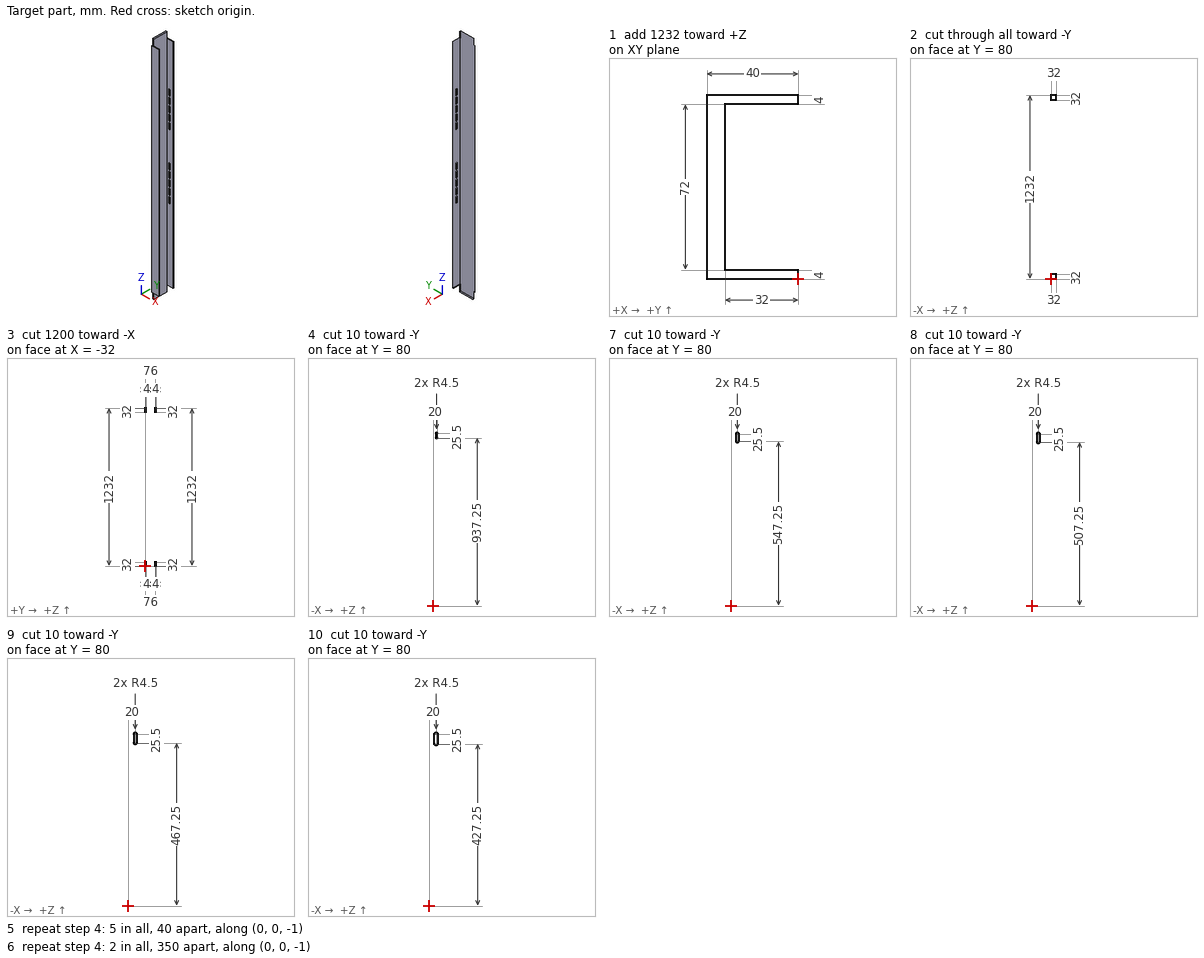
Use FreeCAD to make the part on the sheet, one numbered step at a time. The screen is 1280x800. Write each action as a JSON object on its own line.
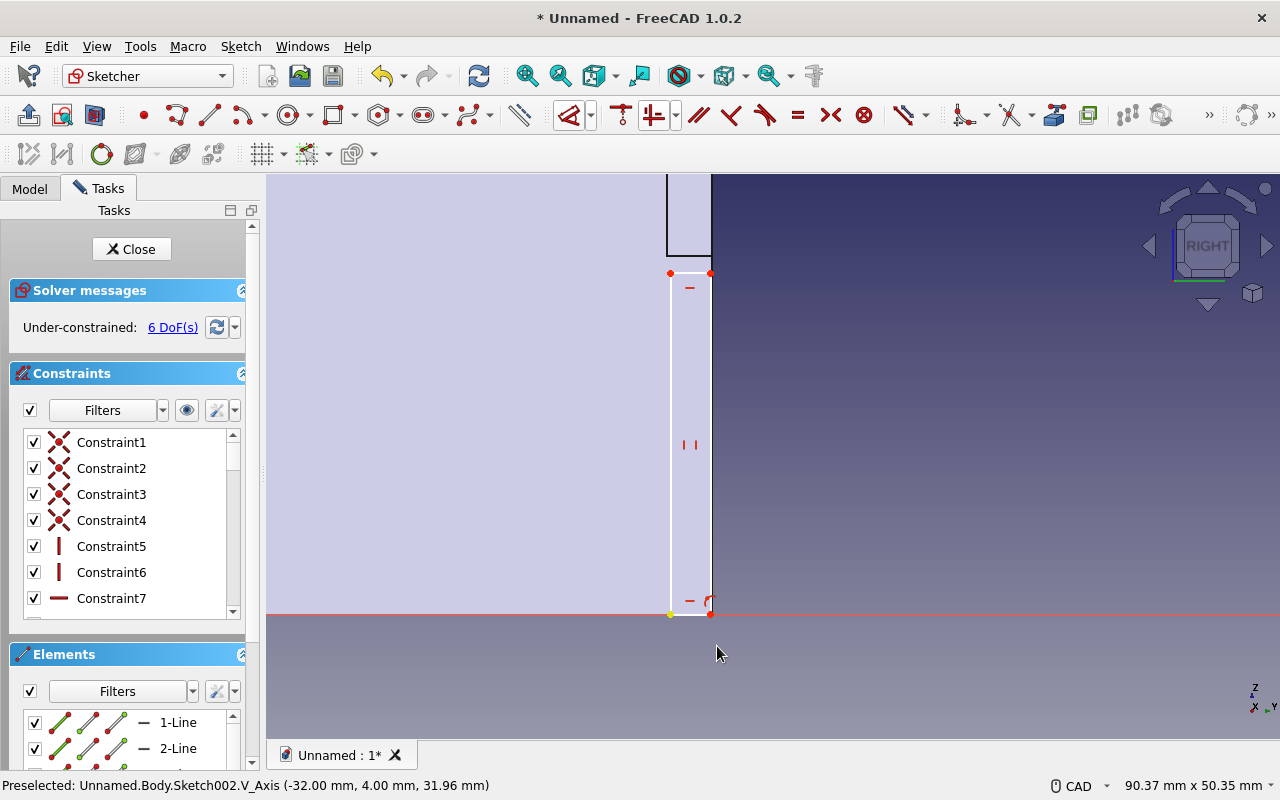
{"action": "left_click", "coordinate": [691, 615]}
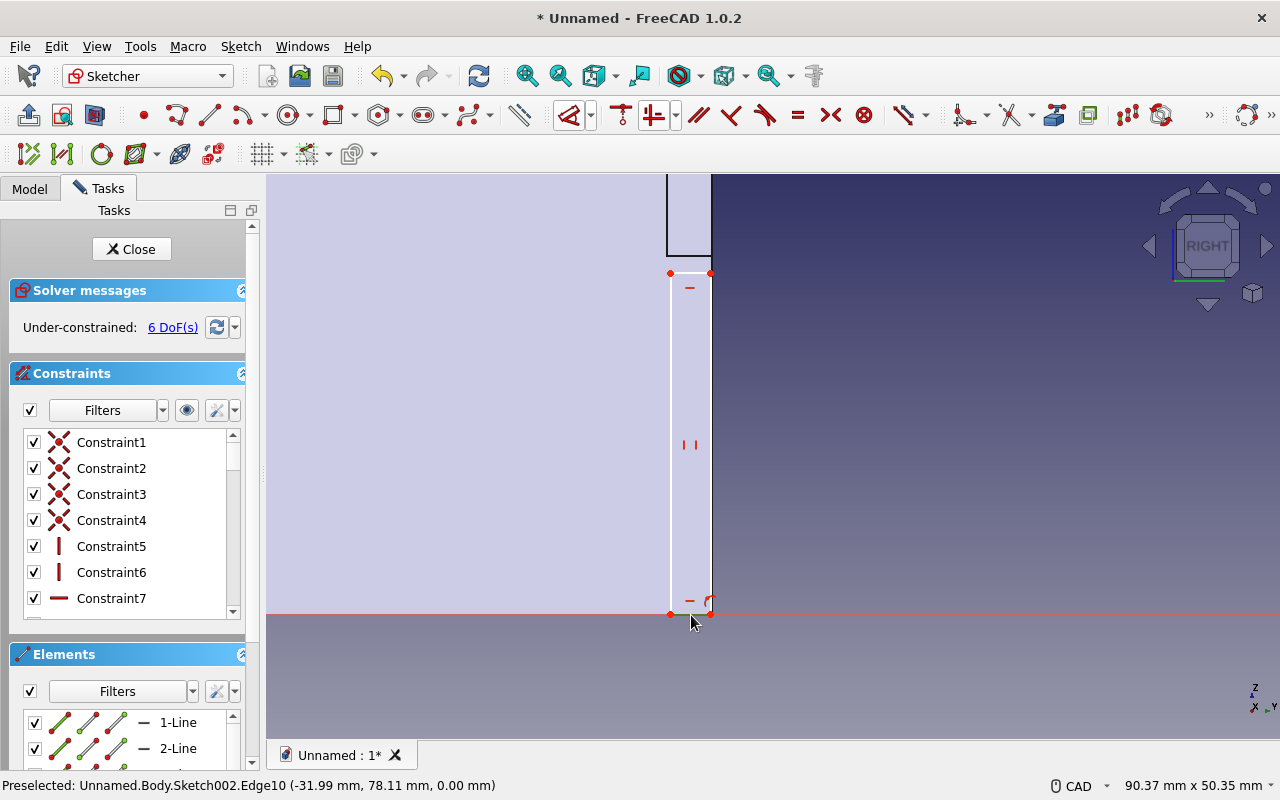
{"action": "key", "text": "l"}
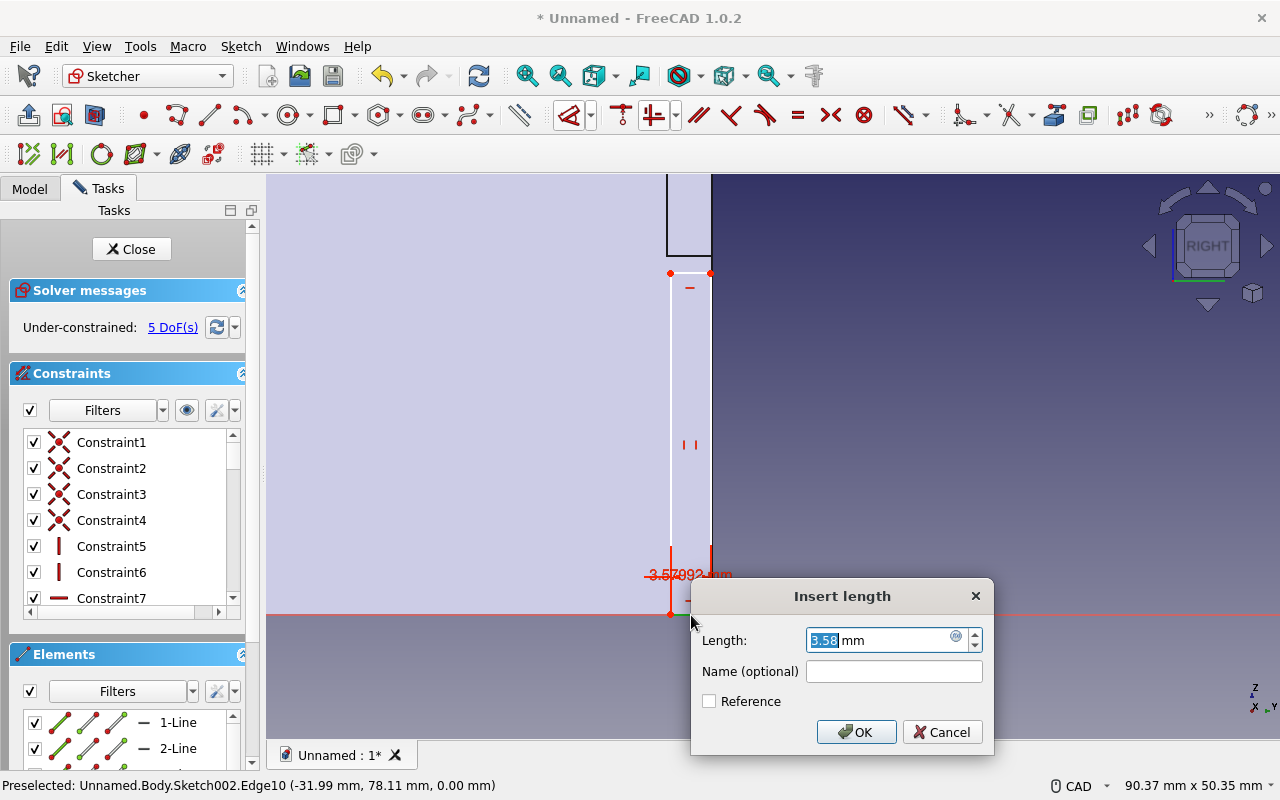
{"action": "type", "text": "4"}
{"action": "key", "text": "Return"}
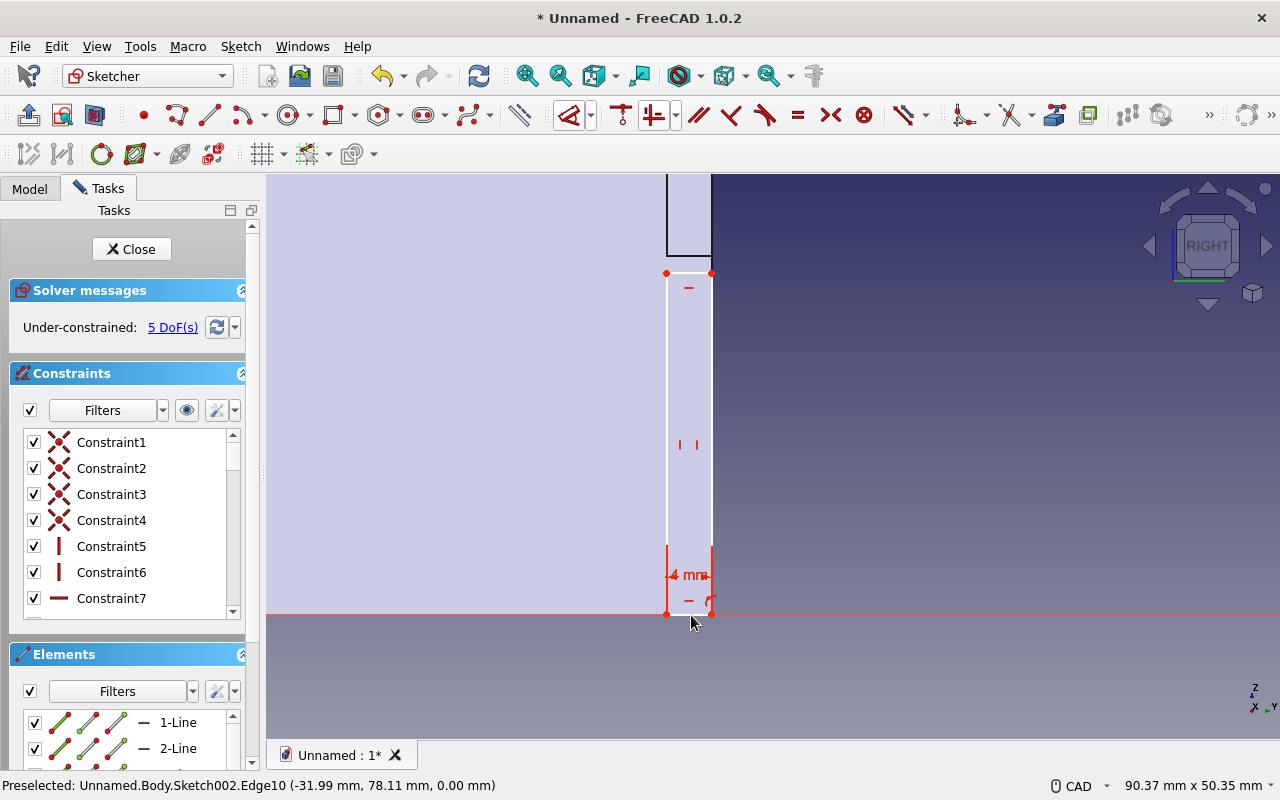
{"action": "scroll", "coordinate": [717, 646], "scroll_direction": "down", "scroll_amount": 18}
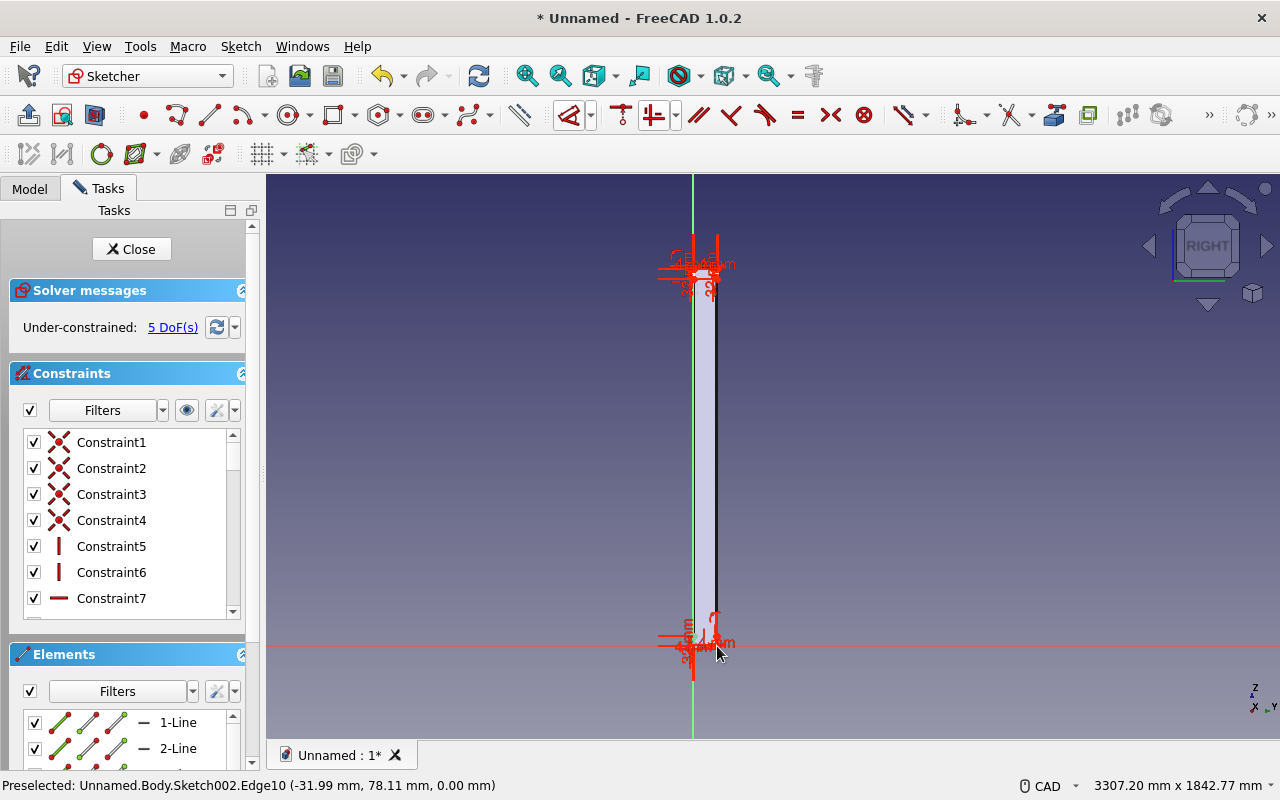
{"action": "scroll", "coordinate": [716, 639], "scroll_direction": "up", "scroll_amount": 13}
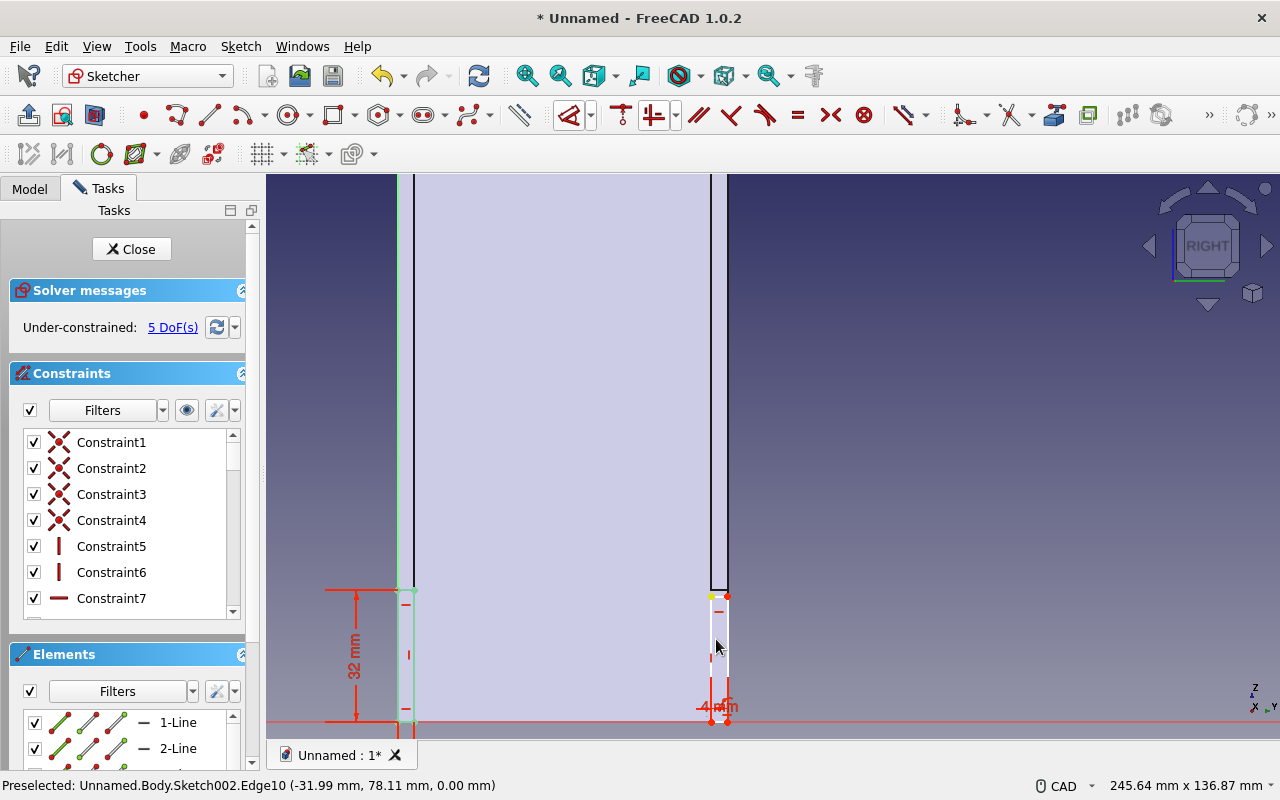
{"action": "left_click", "coordinate": [711, 635]}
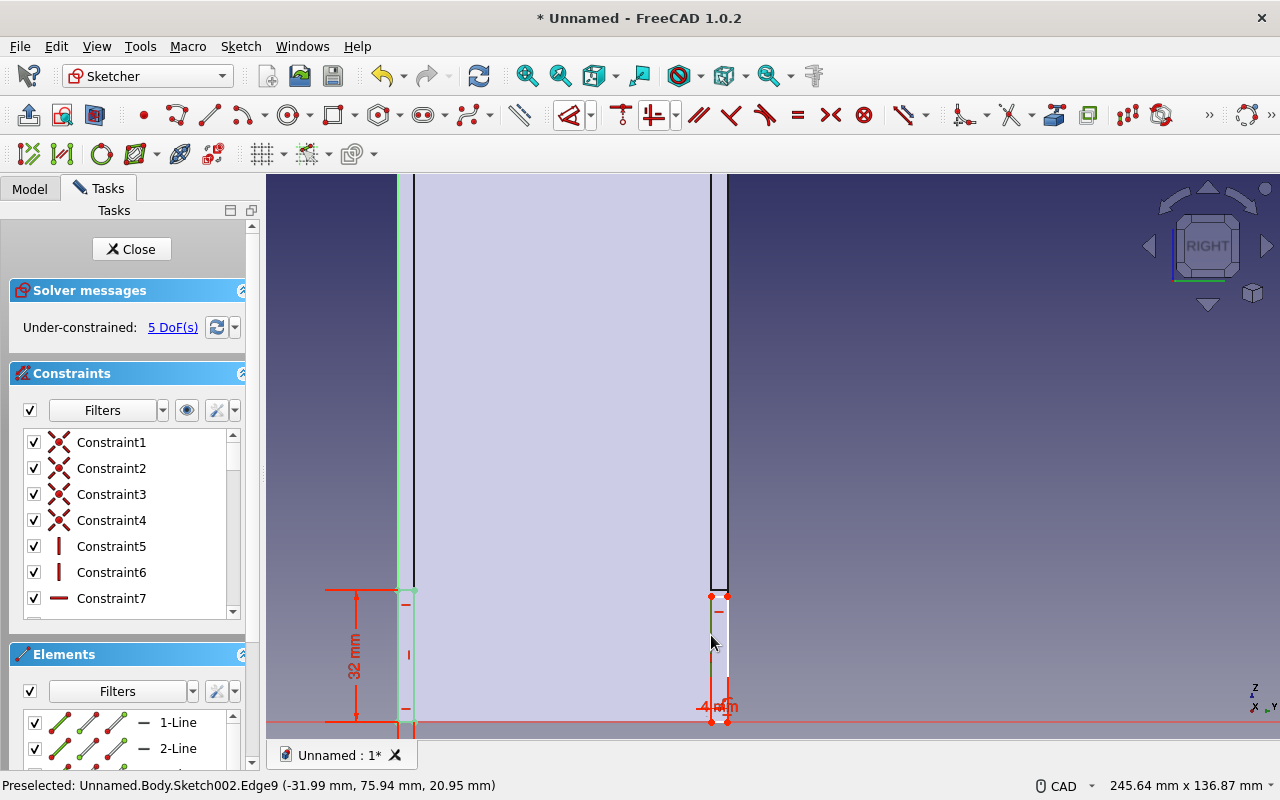
{"action": "key", "text": "i"}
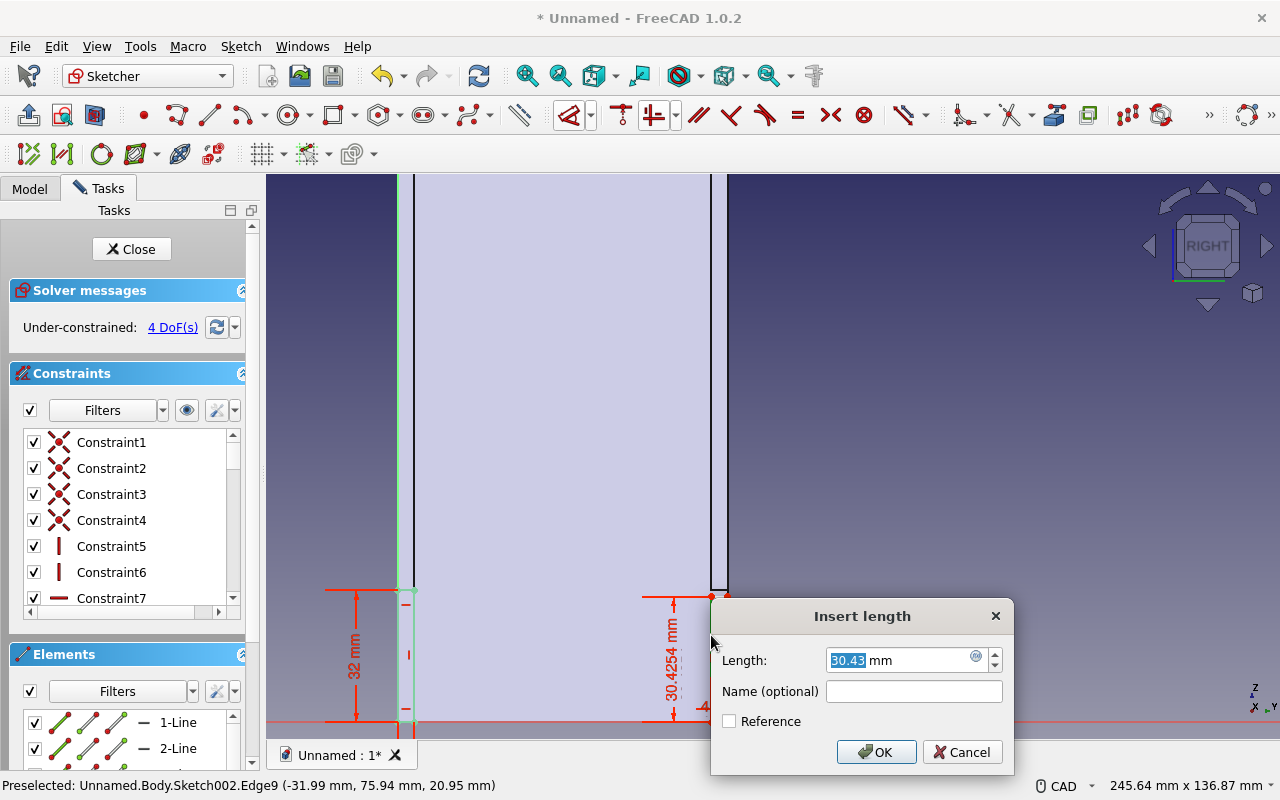
{"action": "type", "text": "32"}
{"action": "key", "text": "Return"}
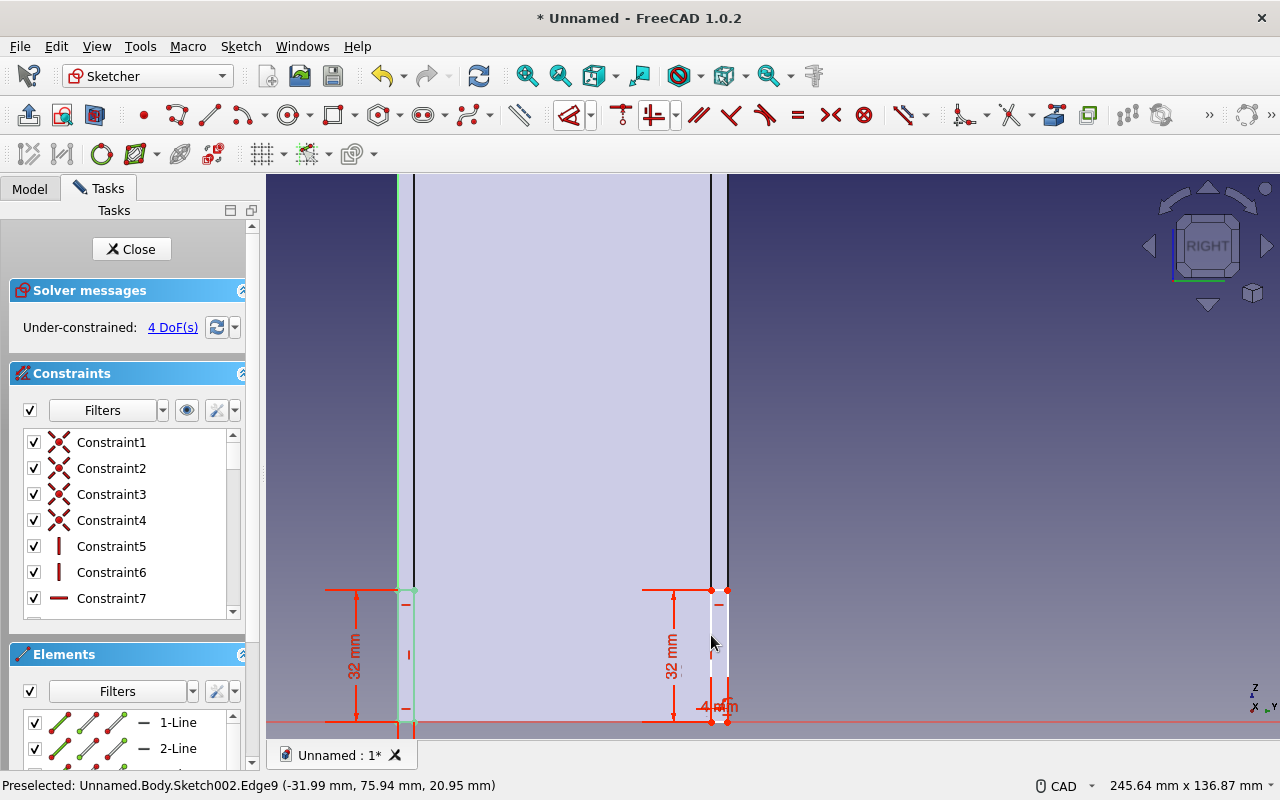
{"action": "scroll", "coordinate": [716, 639], "scroll_direction": "down", "scroll_amount": 13}